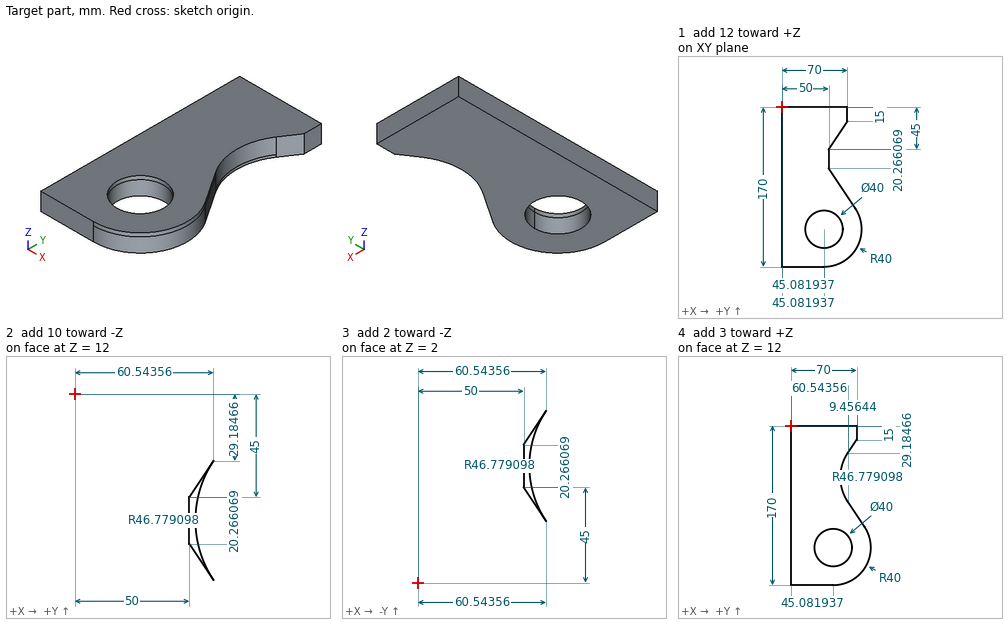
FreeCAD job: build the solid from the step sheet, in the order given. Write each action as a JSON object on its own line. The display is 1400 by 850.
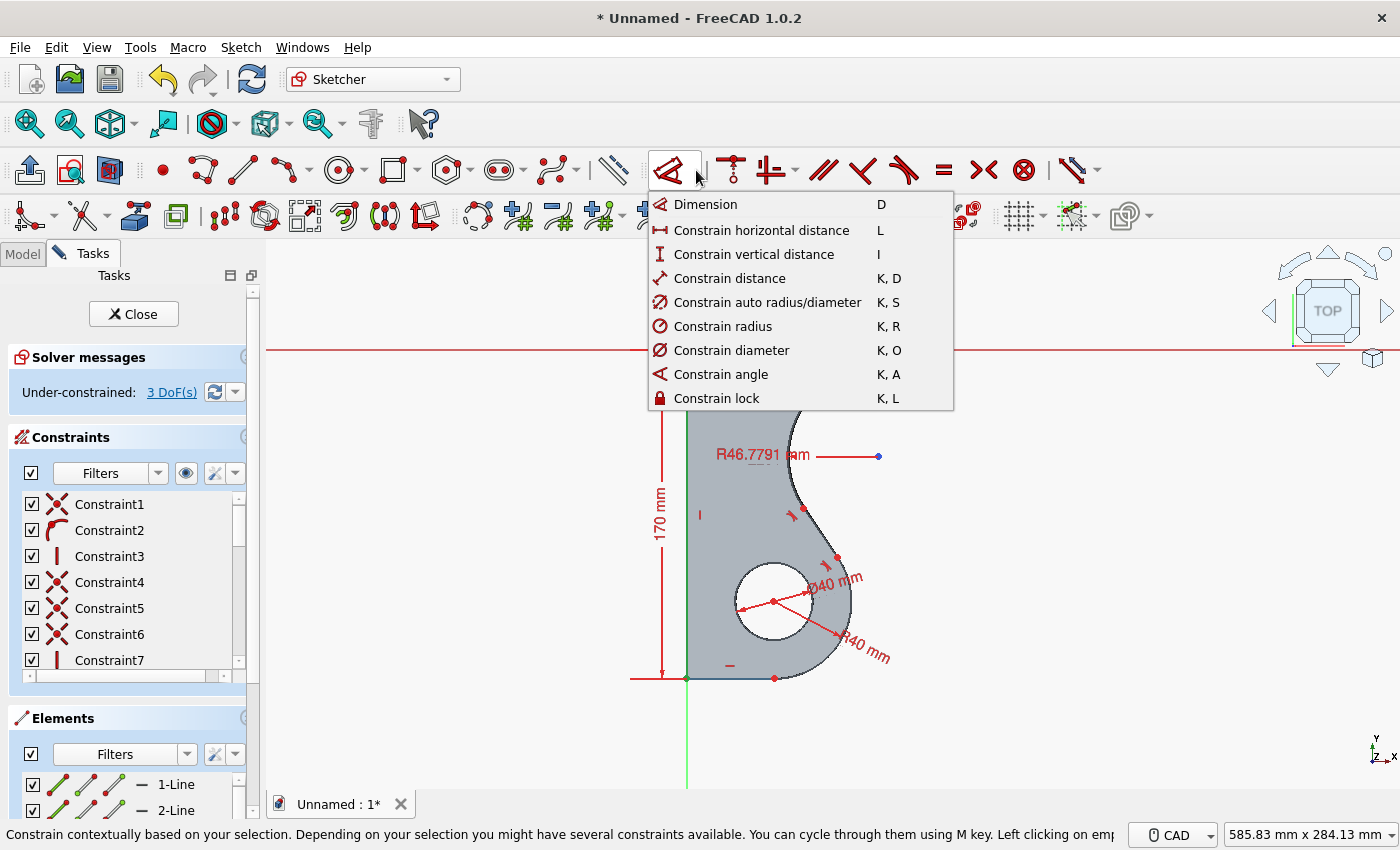
{"action": "left_click", "coordinate": [801, 230]}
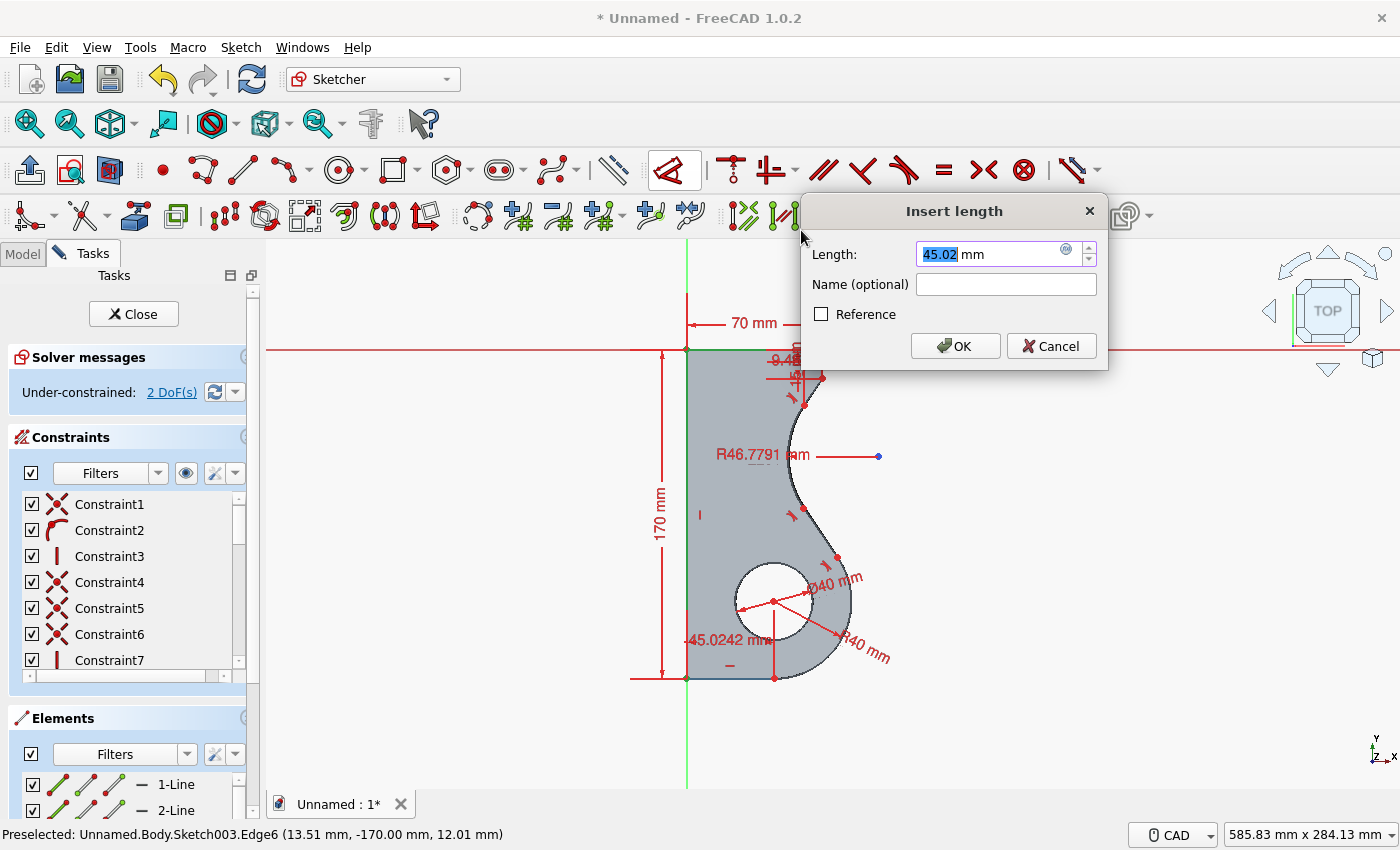
{"action": "type", "text": "45.081937"}
{"action": "key", "text": "Return"}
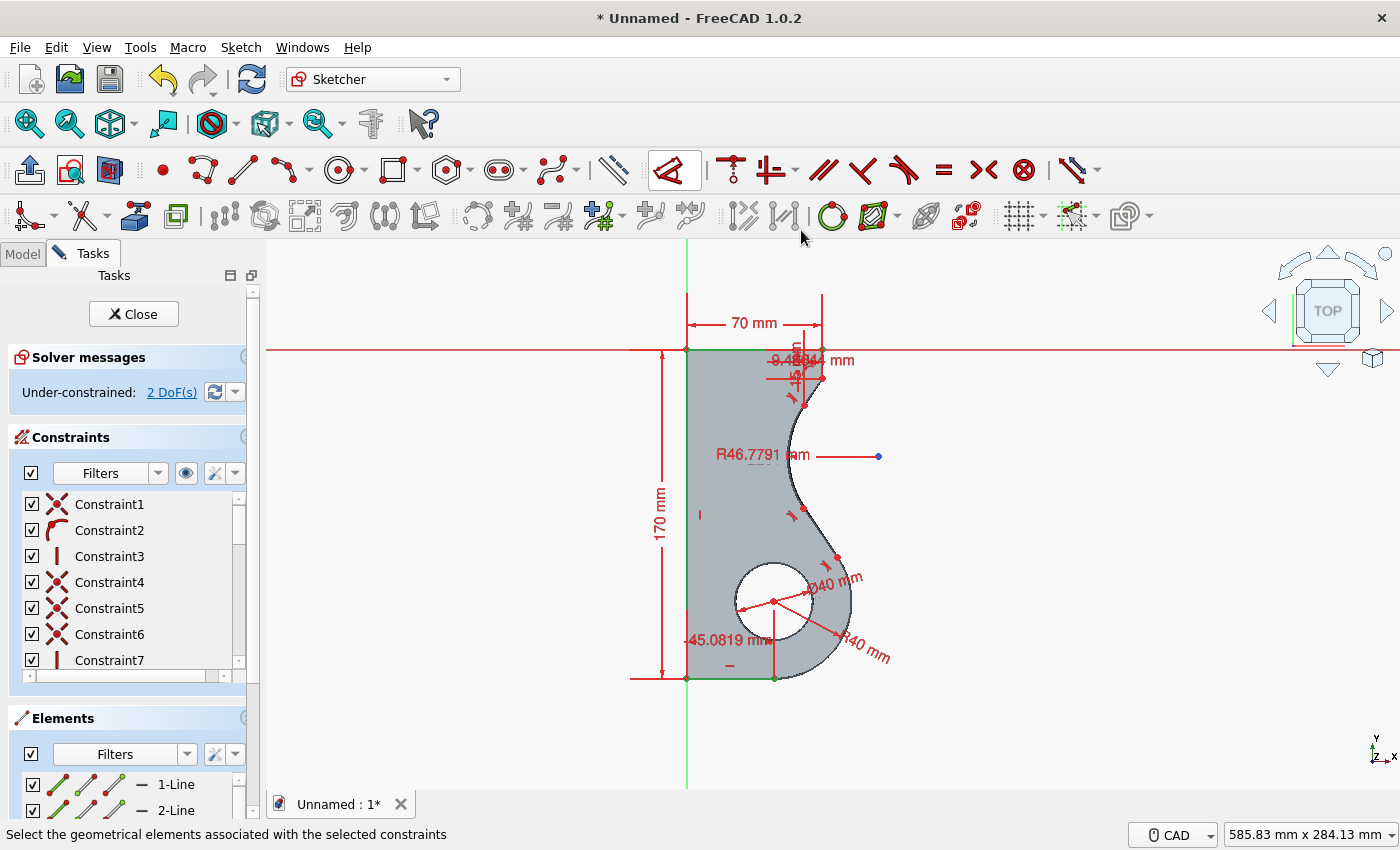
{"action": "left_click", "coordinate": [804, 508]}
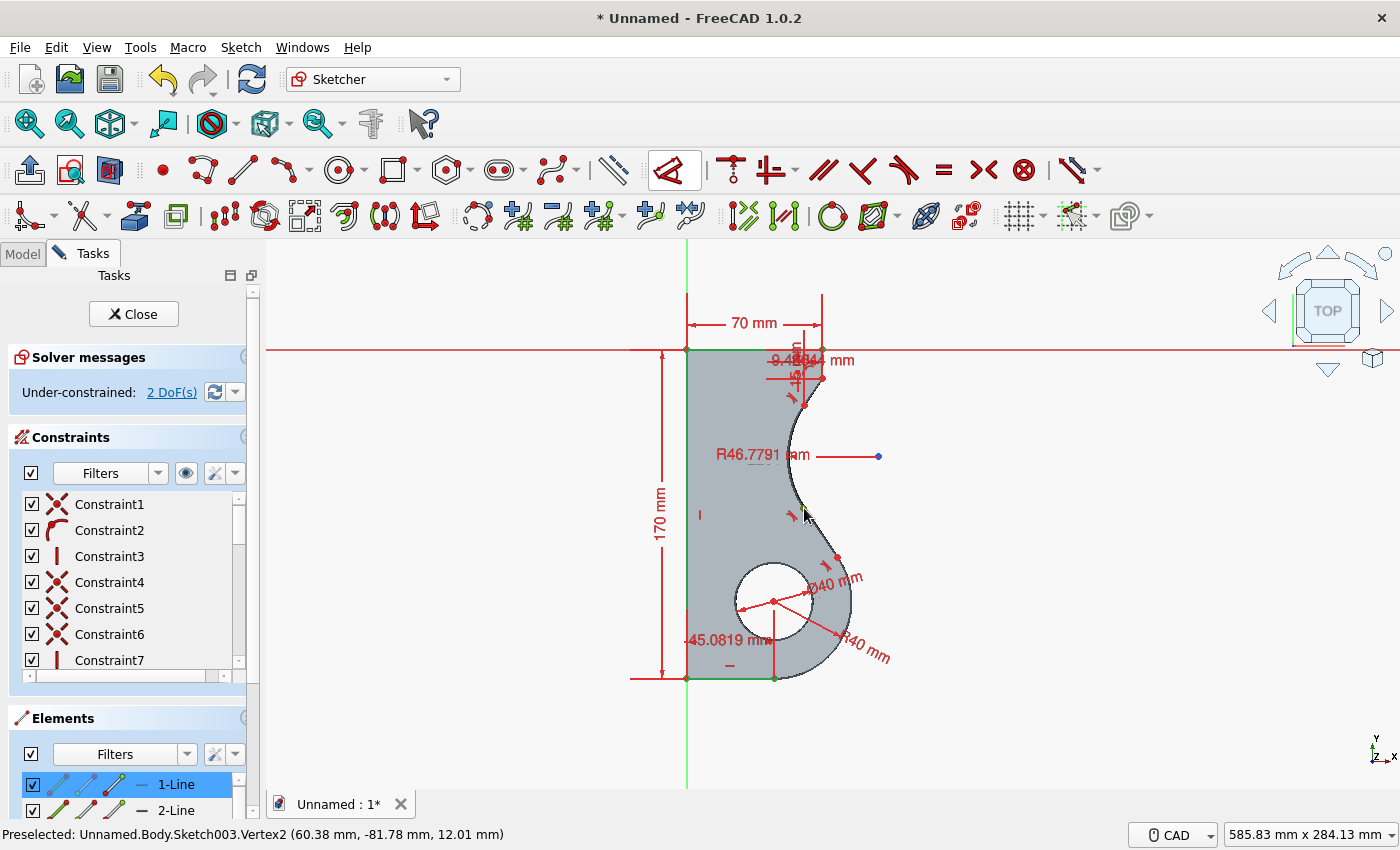
{"action": "key", "text": "l"}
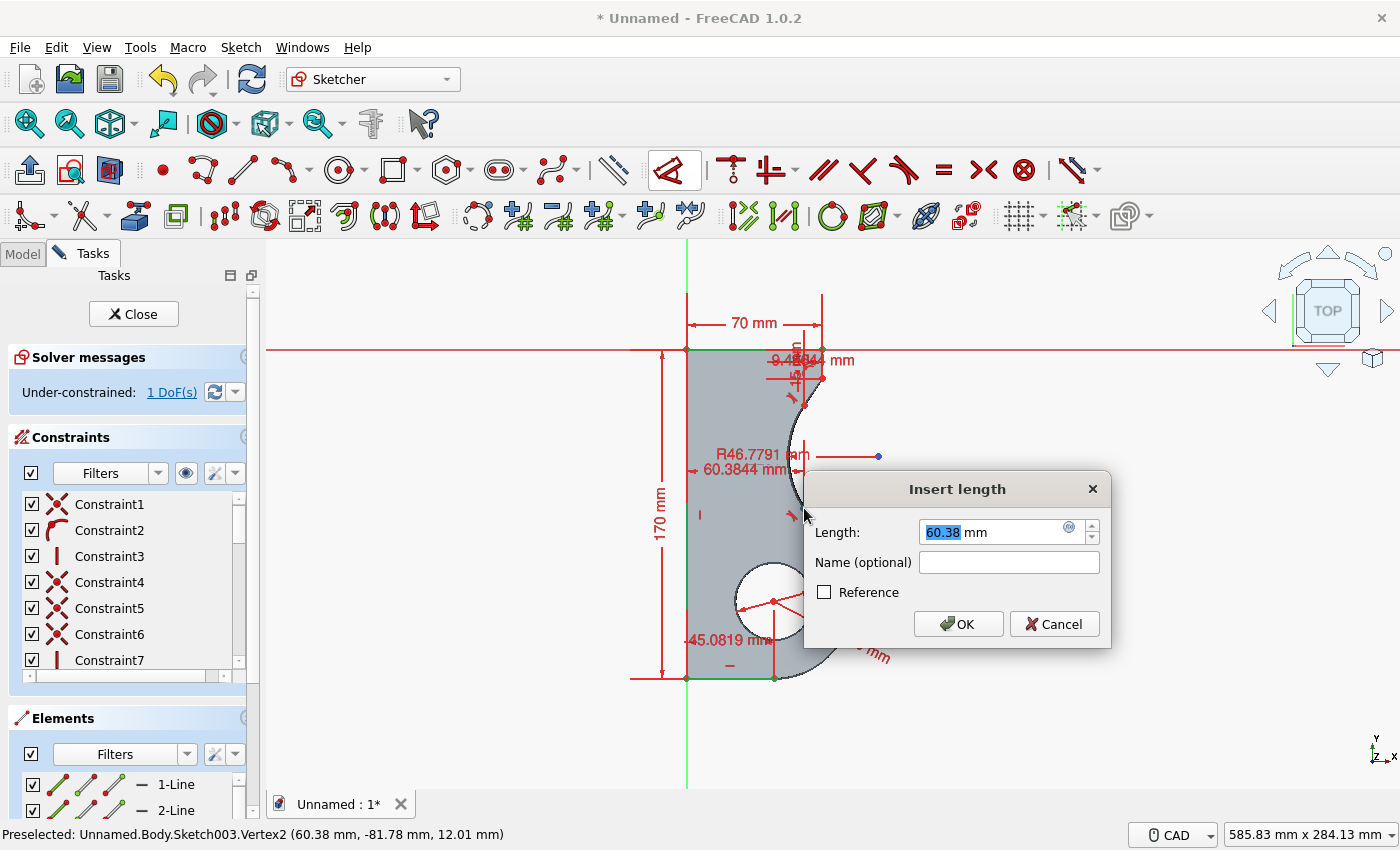
{"action": "type", "text": "60.54356"}
{"action": "key", "text": "Return"}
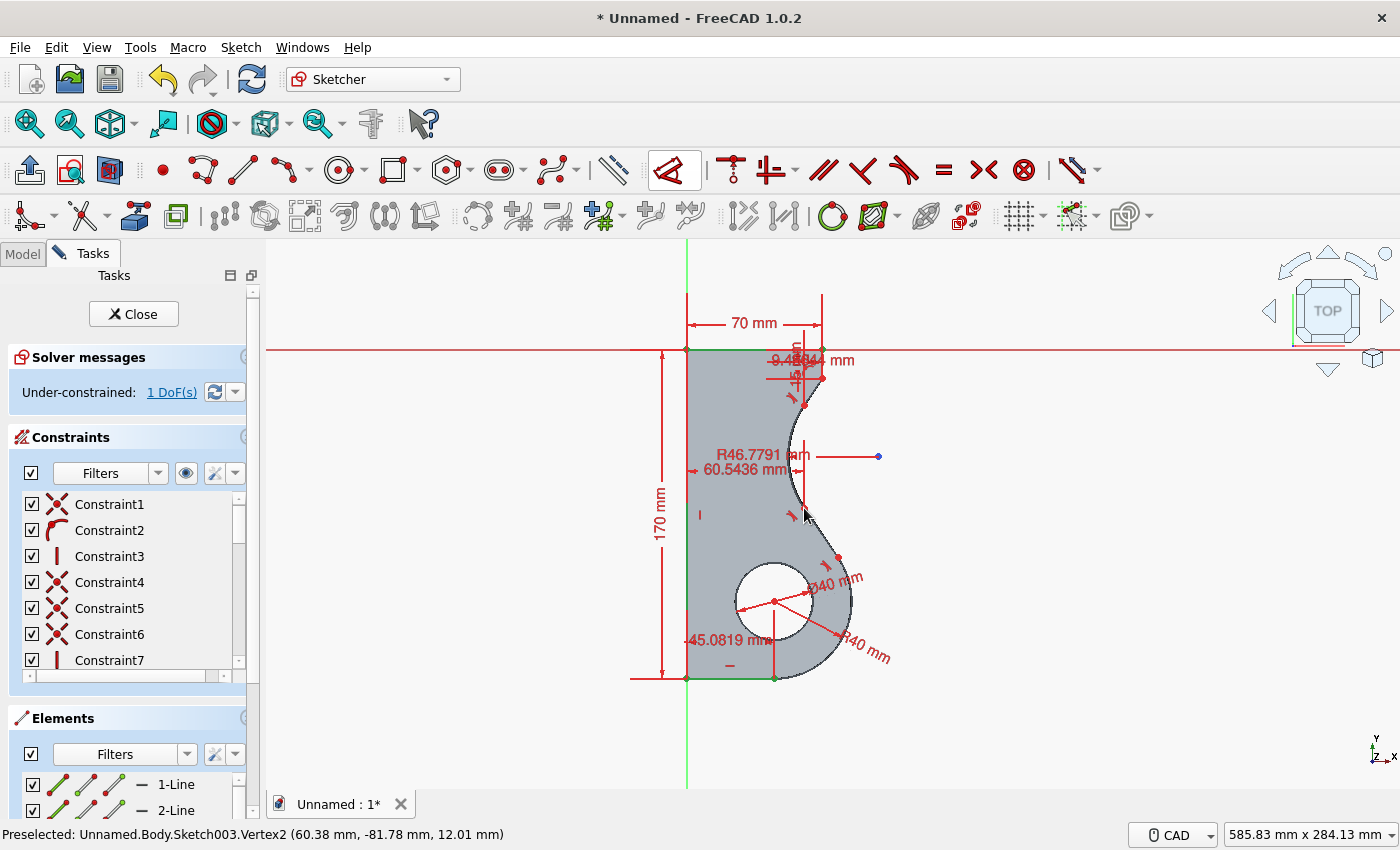
{"action": "left_click", "coordinate": [804, 405]}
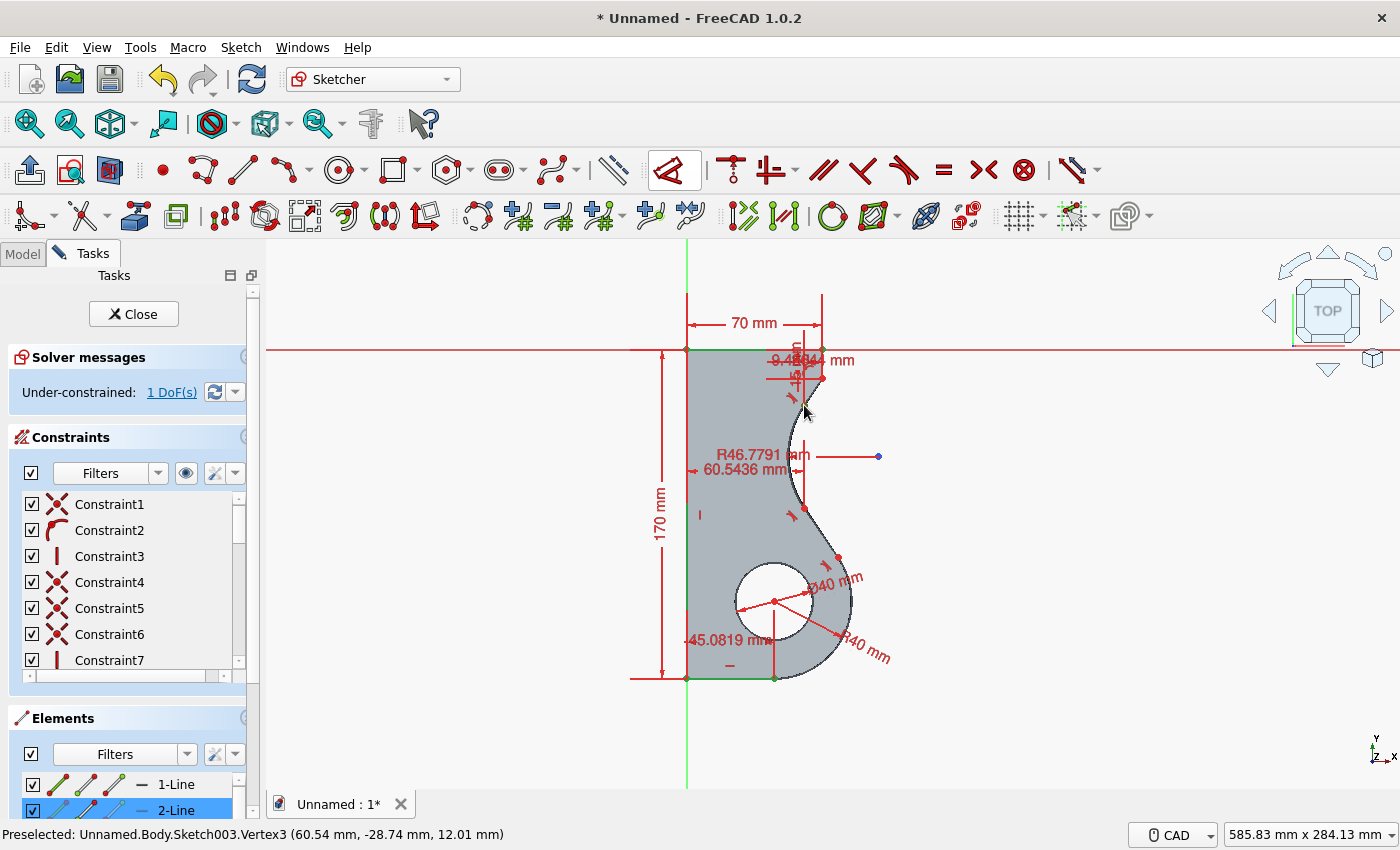
{"action": "left_click", "coordinate": [696, 170]}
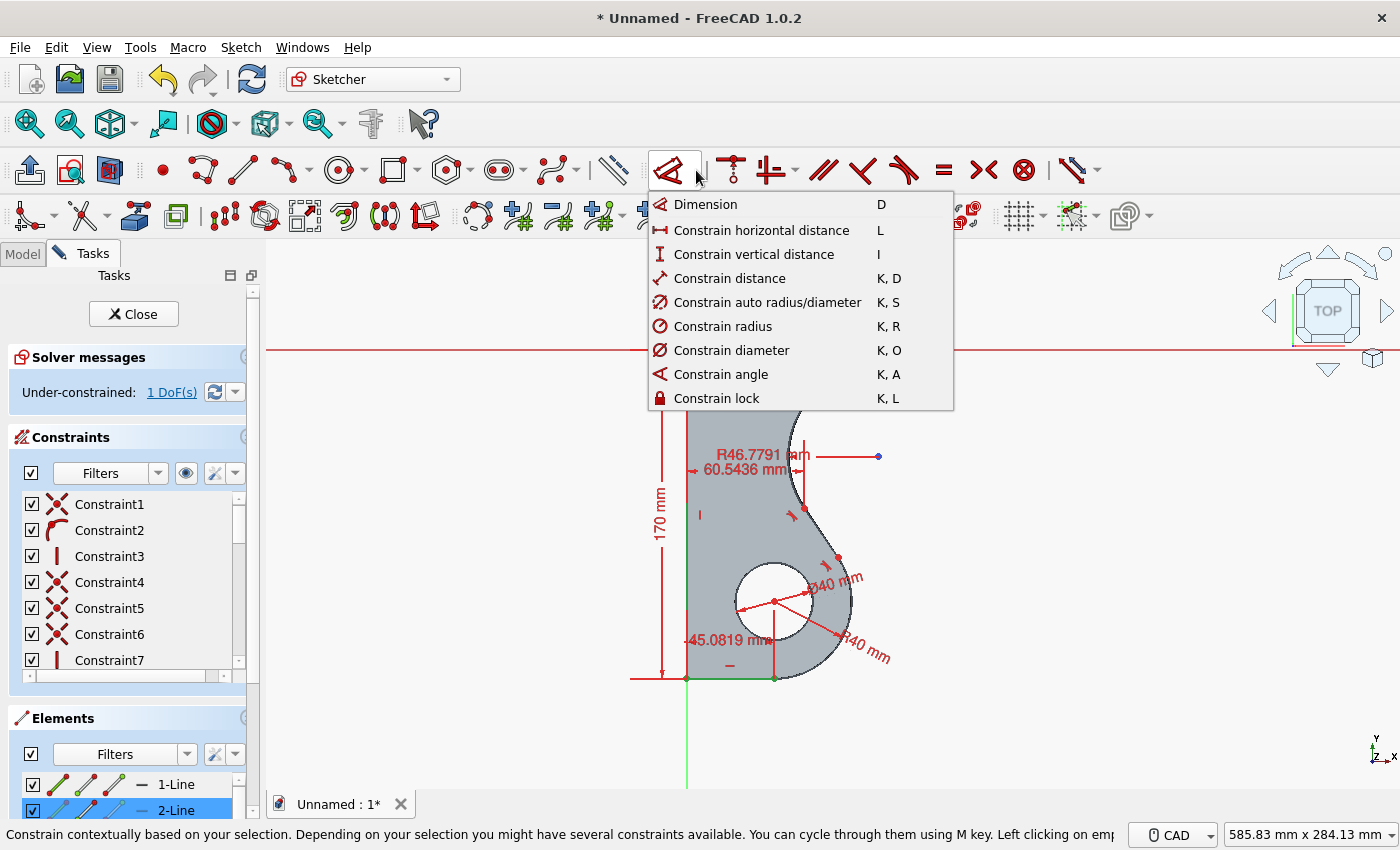
{"action": "left_click", "coordinate": [801, 254]}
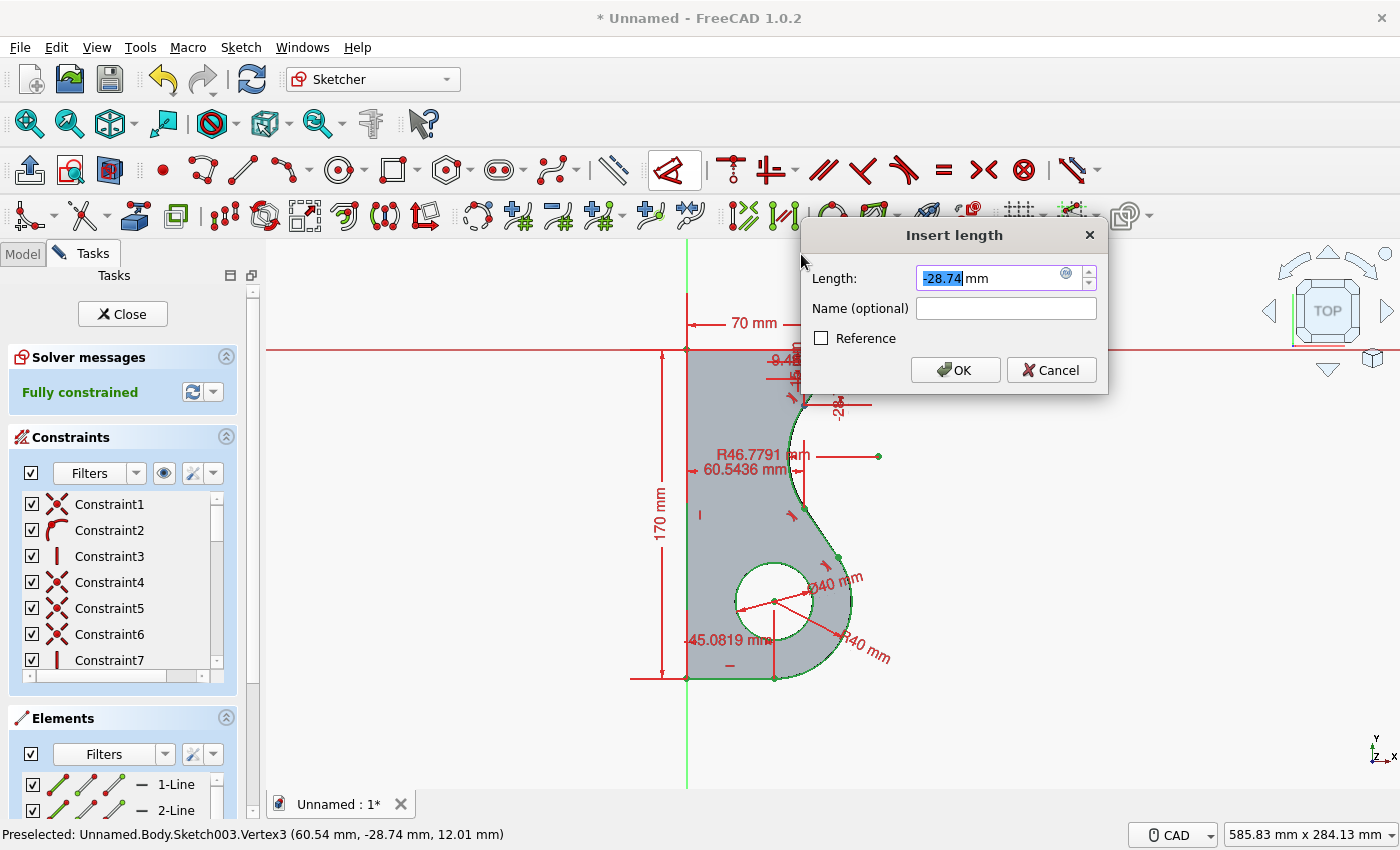
{"action": "type", "text": "-29.18466"}
{"action": "key", "text": "Return"}